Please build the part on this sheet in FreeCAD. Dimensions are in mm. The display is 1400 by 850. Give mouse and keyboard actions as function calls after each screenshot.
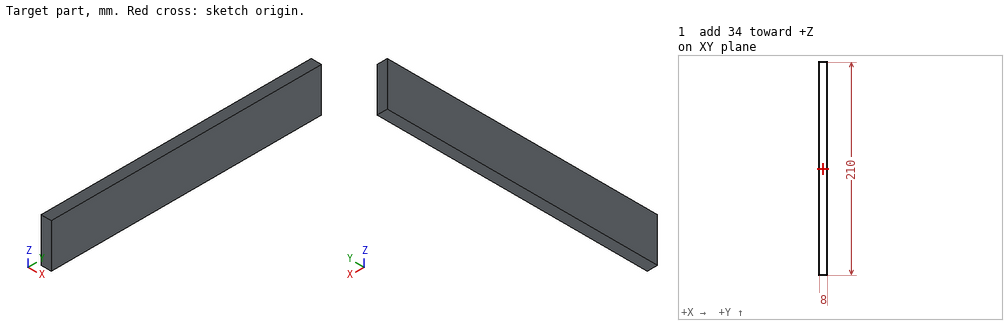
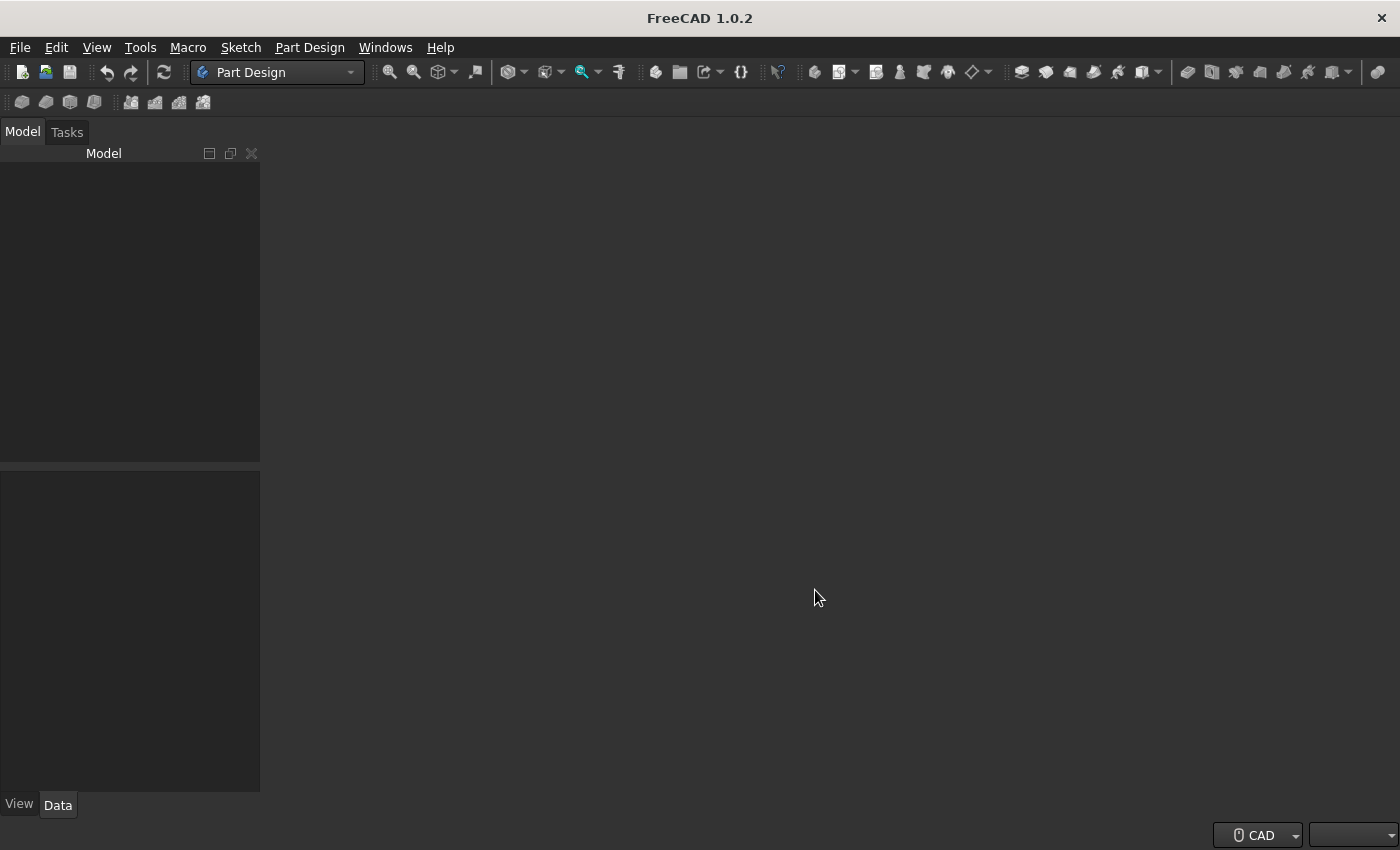
click(22, 72)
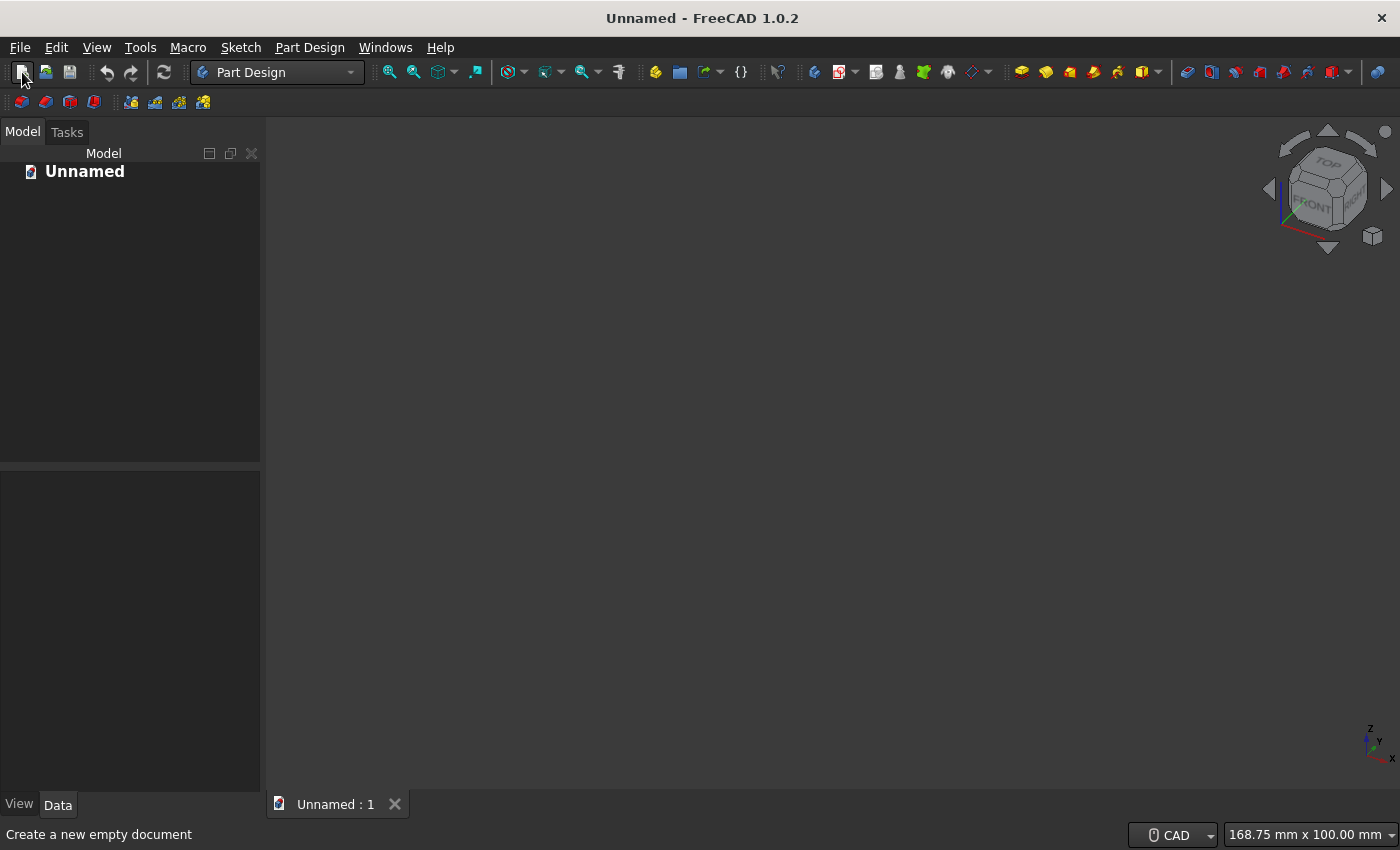
click(840, 72)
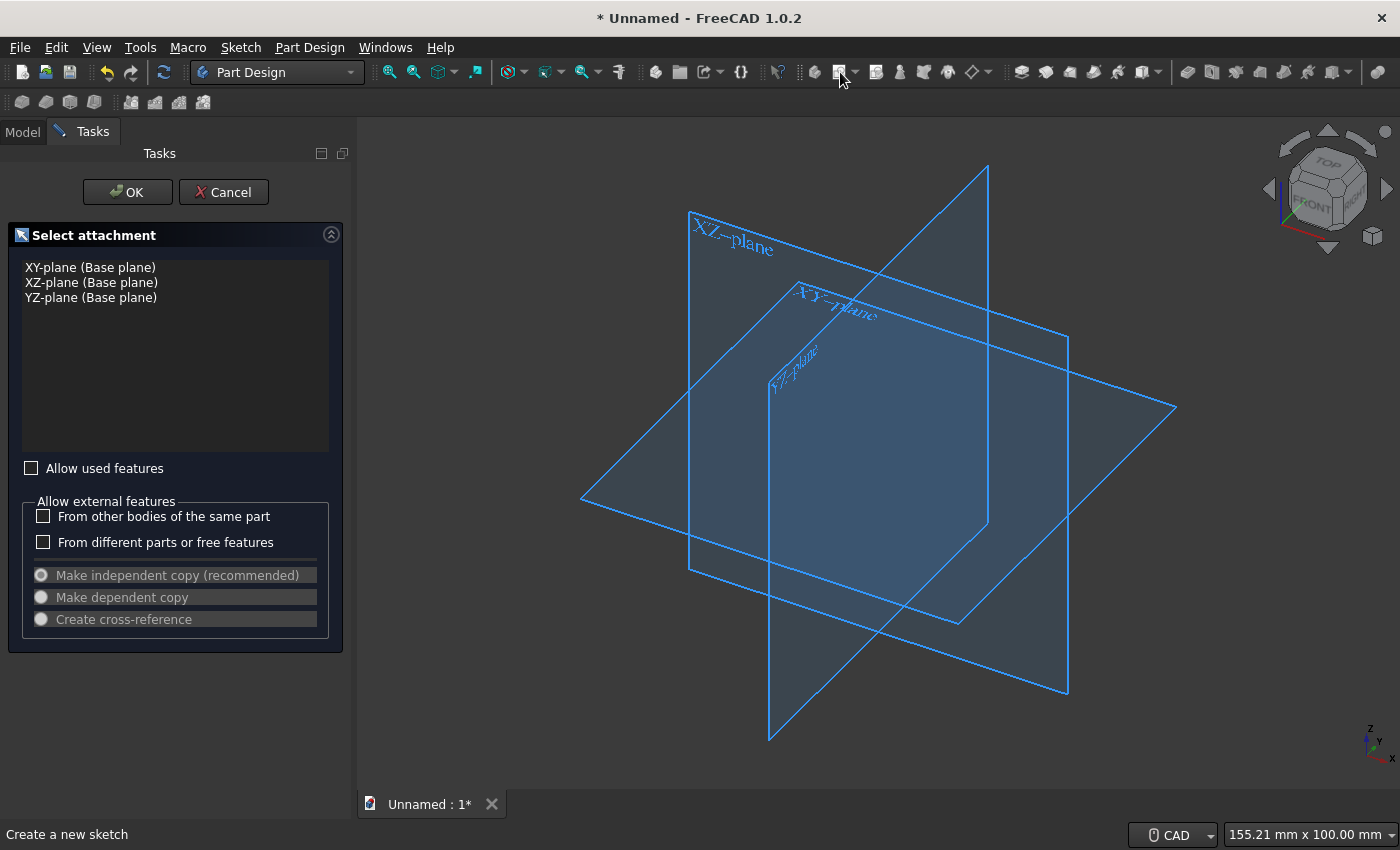
click(82, 268)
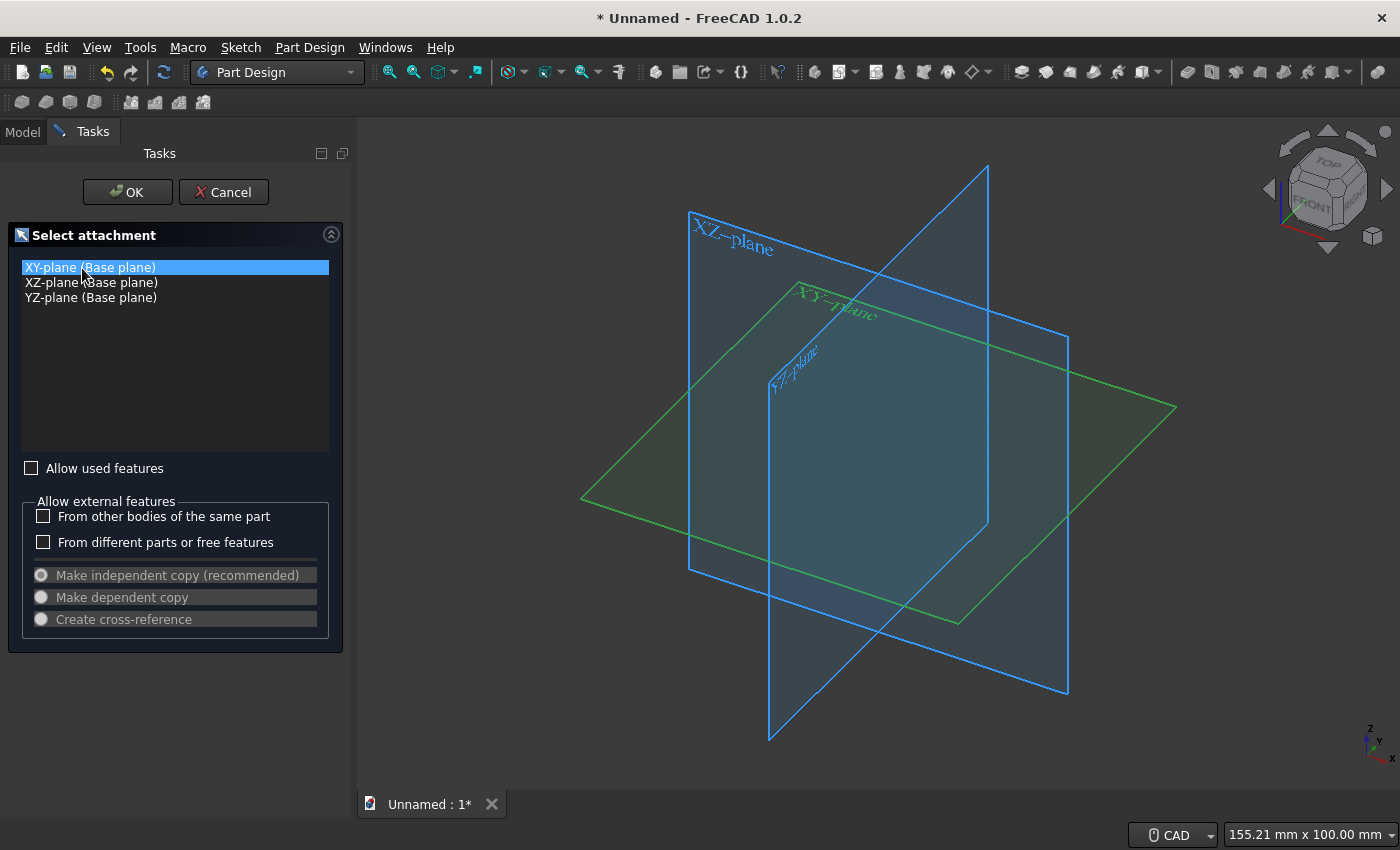
click(128, 192)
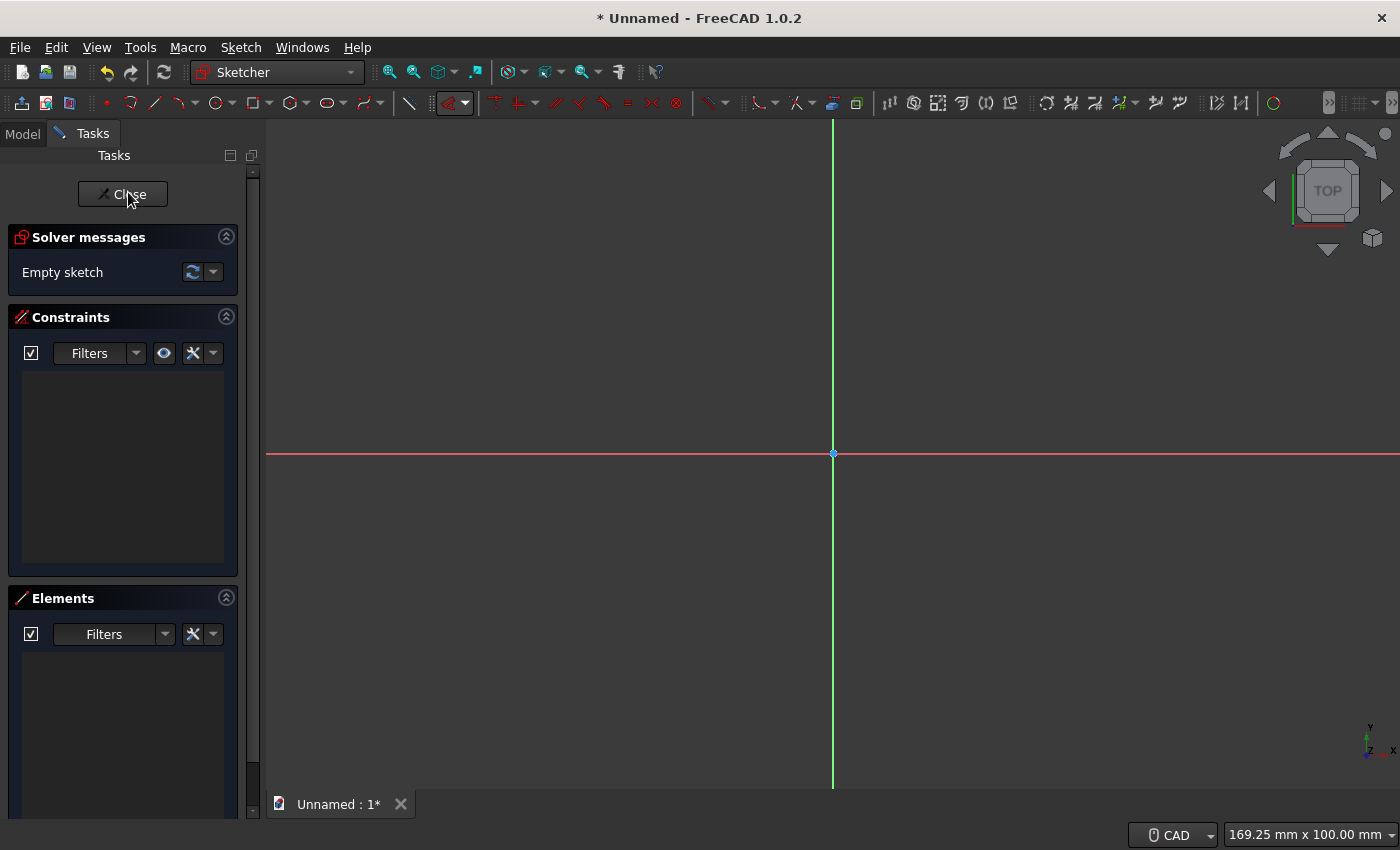
scroll(735, 454, down, 6)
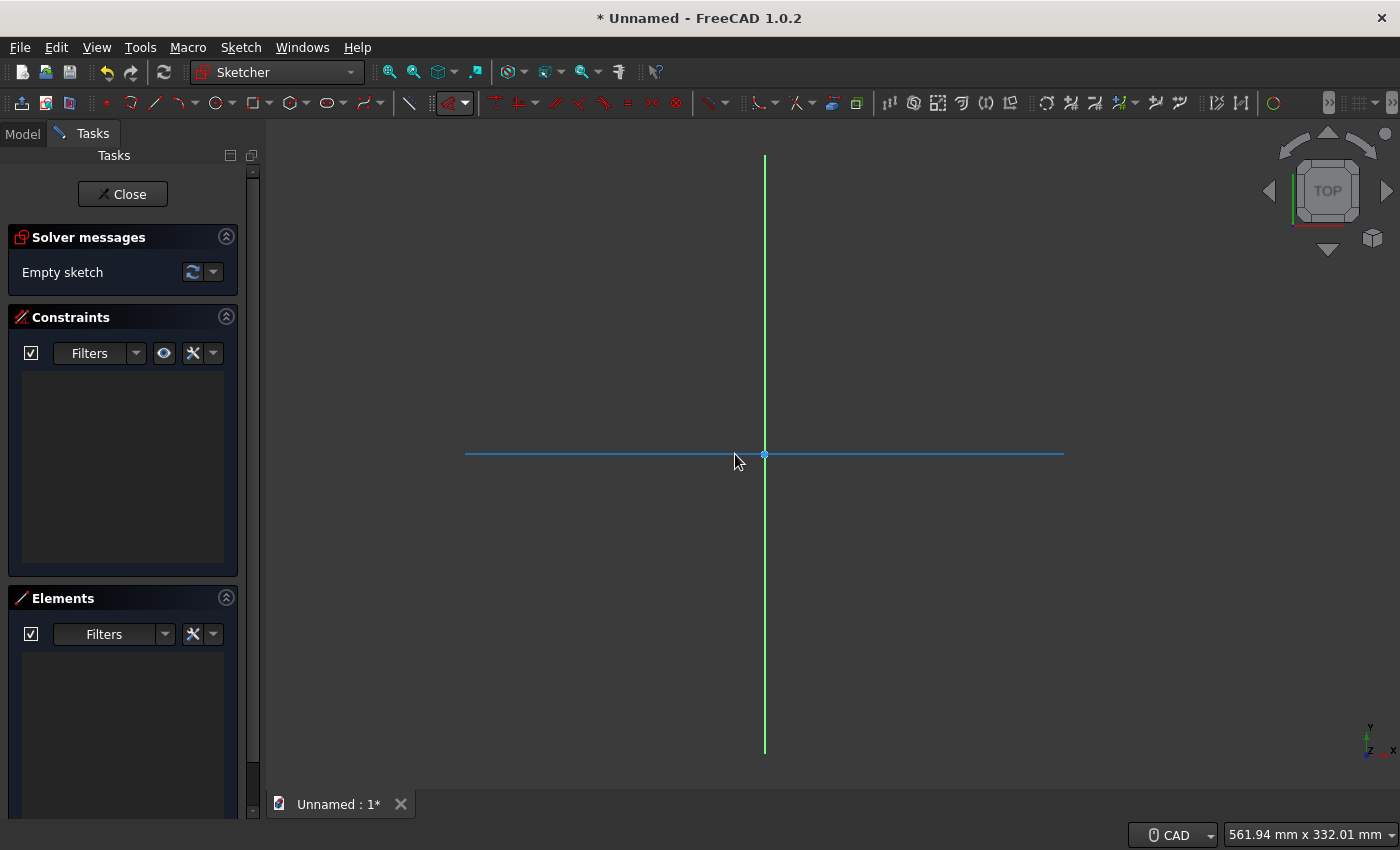
key(g)
key(v)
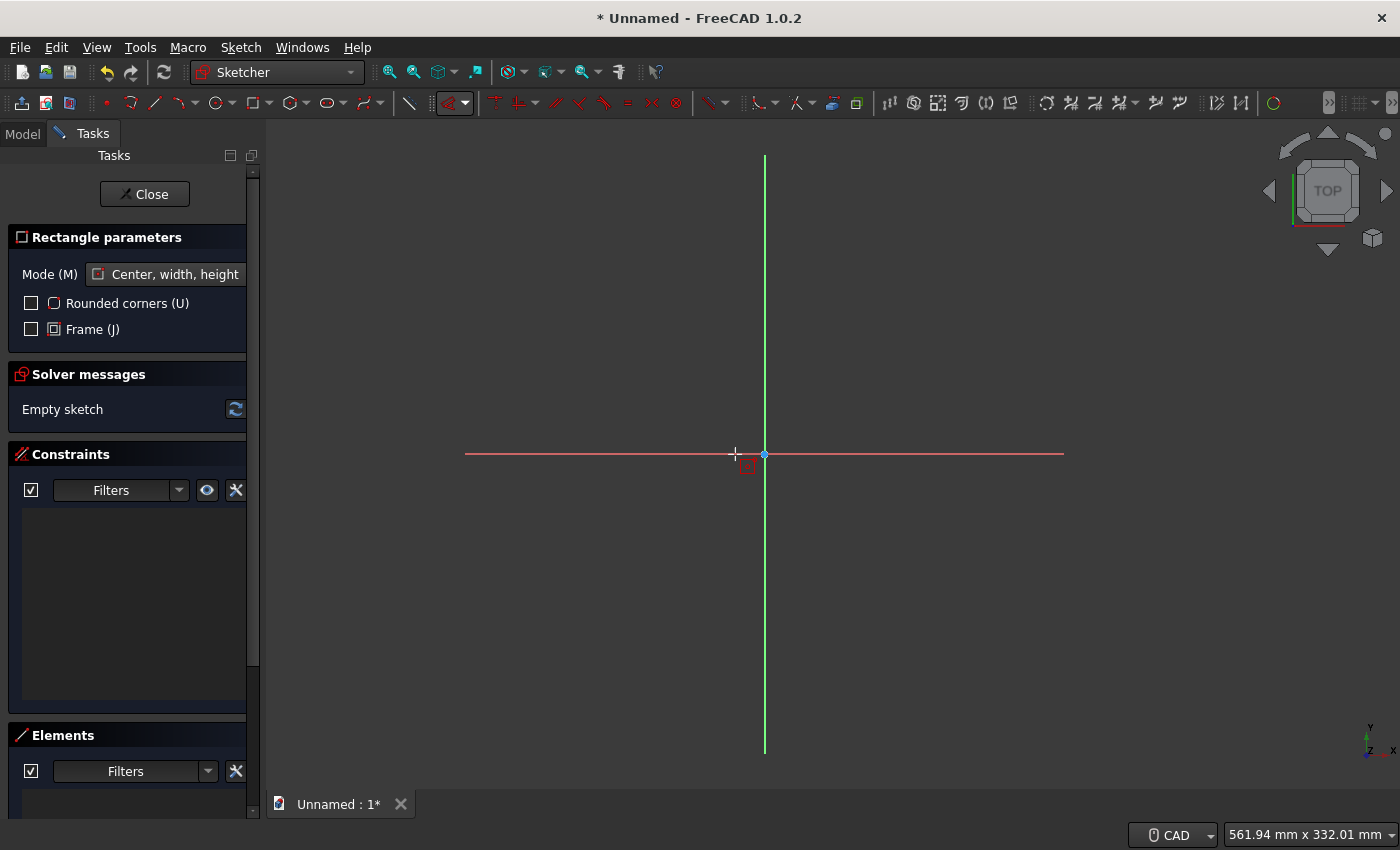
scroll(765, 454, up, 4)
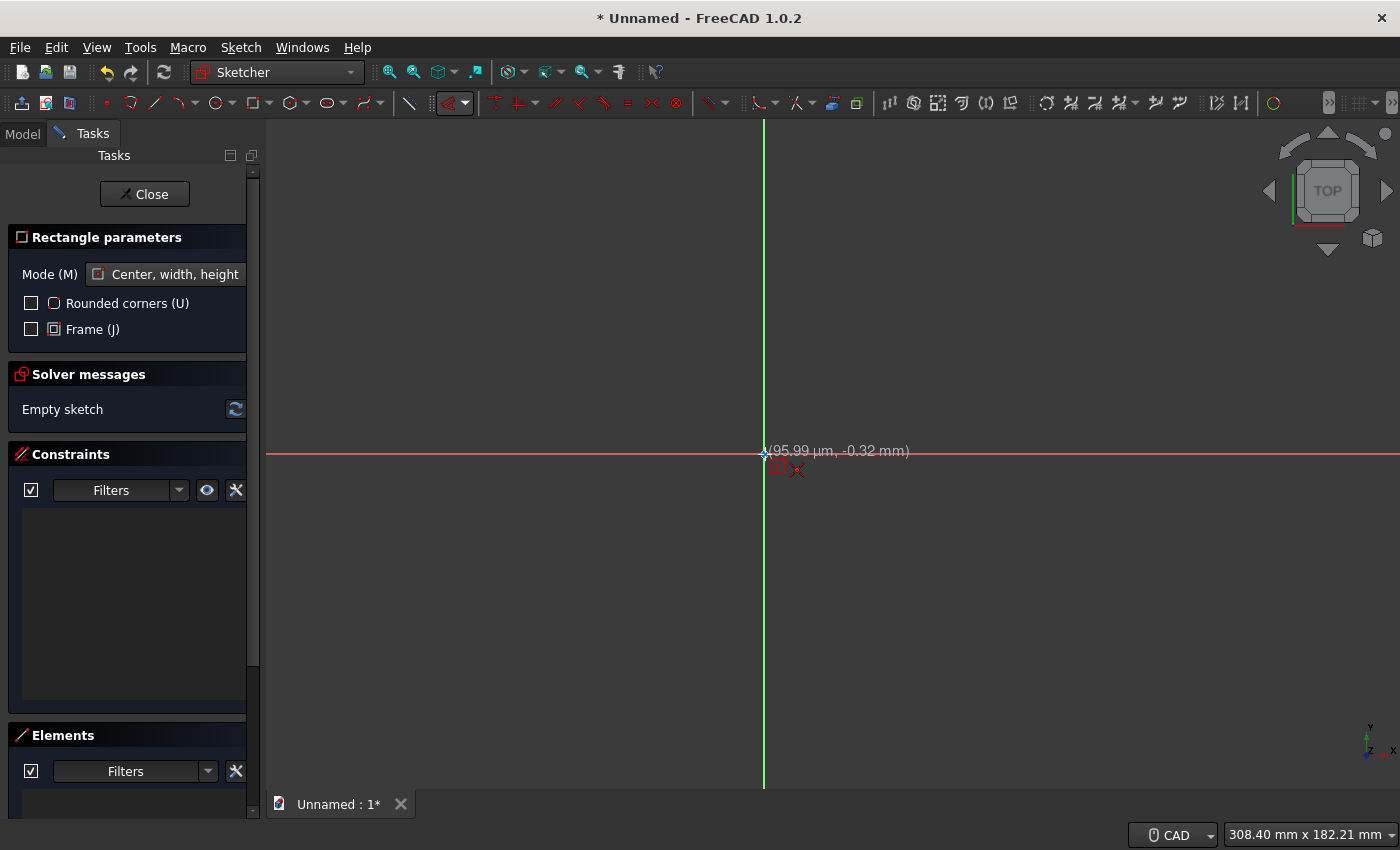
click(764, 454)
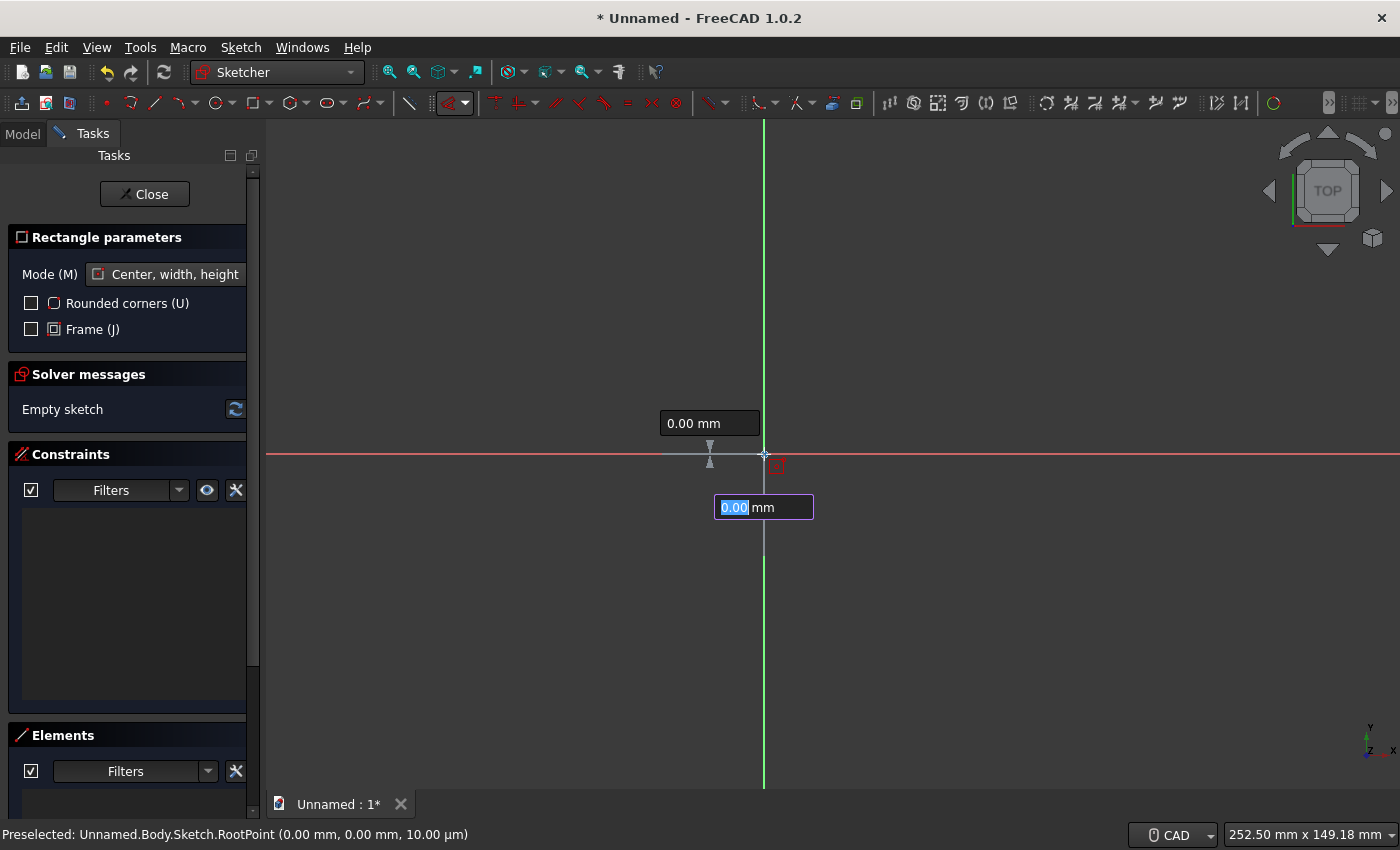
scroll(765, 454, down, 4)